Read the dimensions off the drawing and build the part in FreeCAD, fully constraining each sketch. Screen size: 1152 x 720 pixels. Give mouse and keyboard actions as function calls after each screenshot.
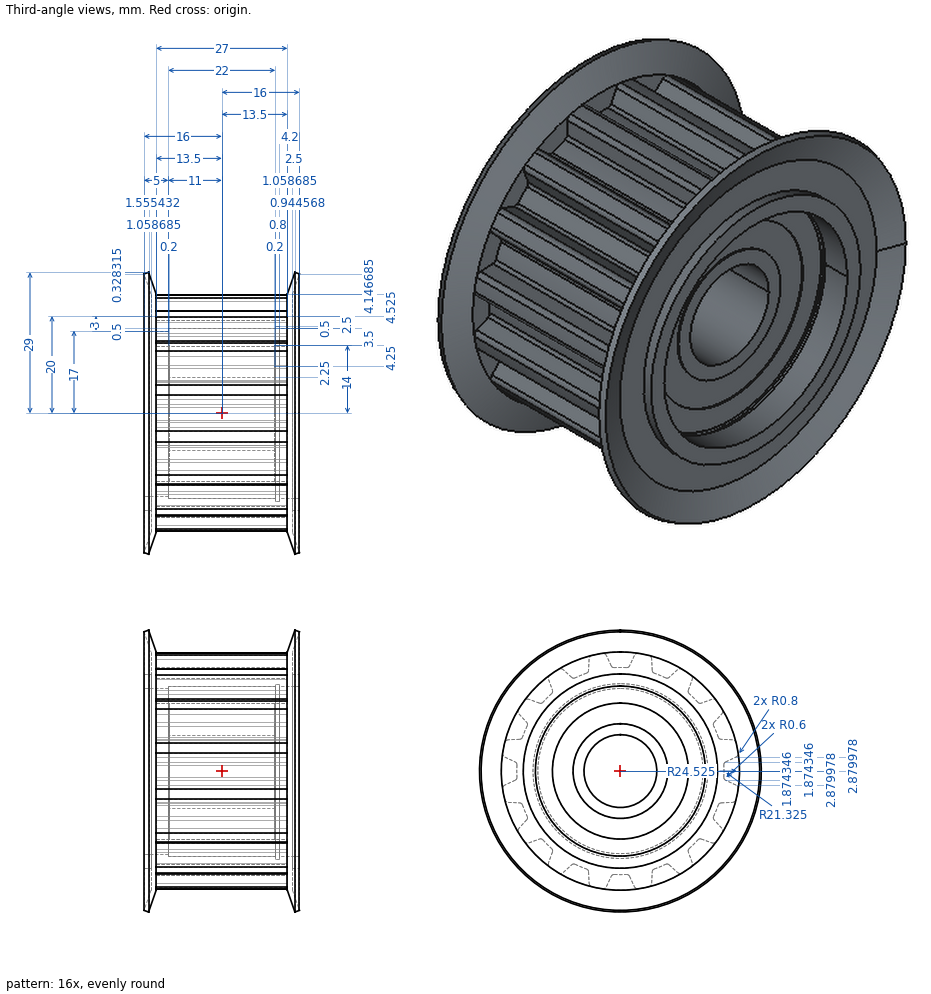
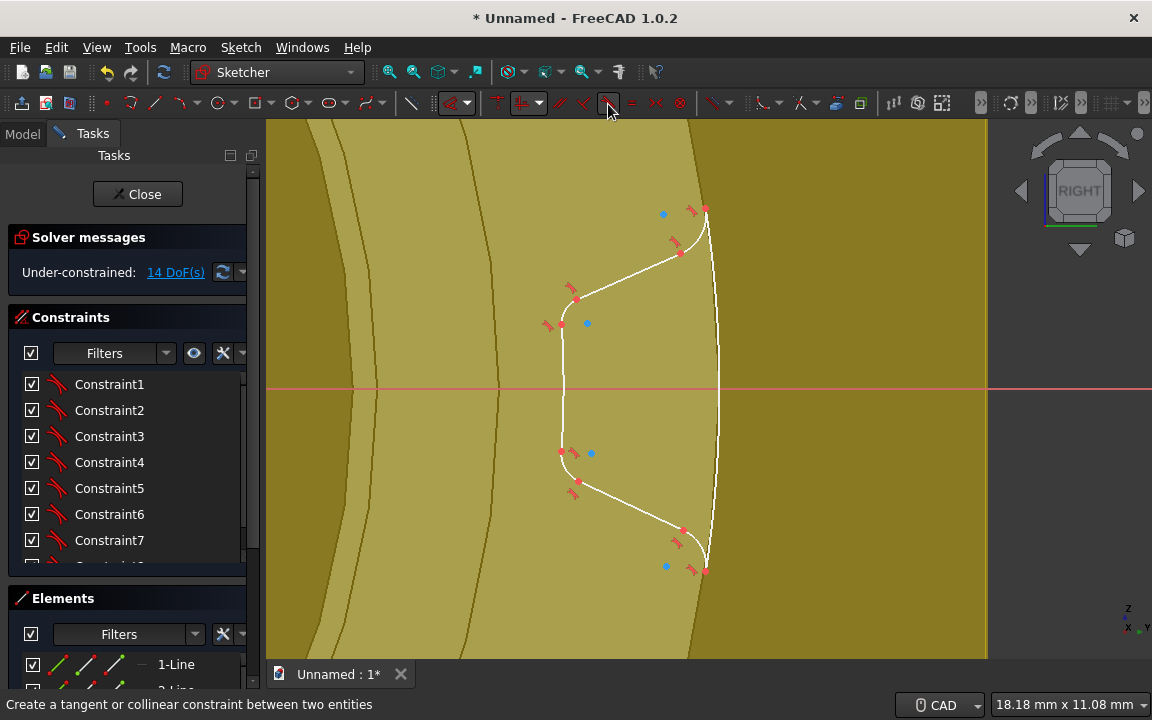
click(563, 414)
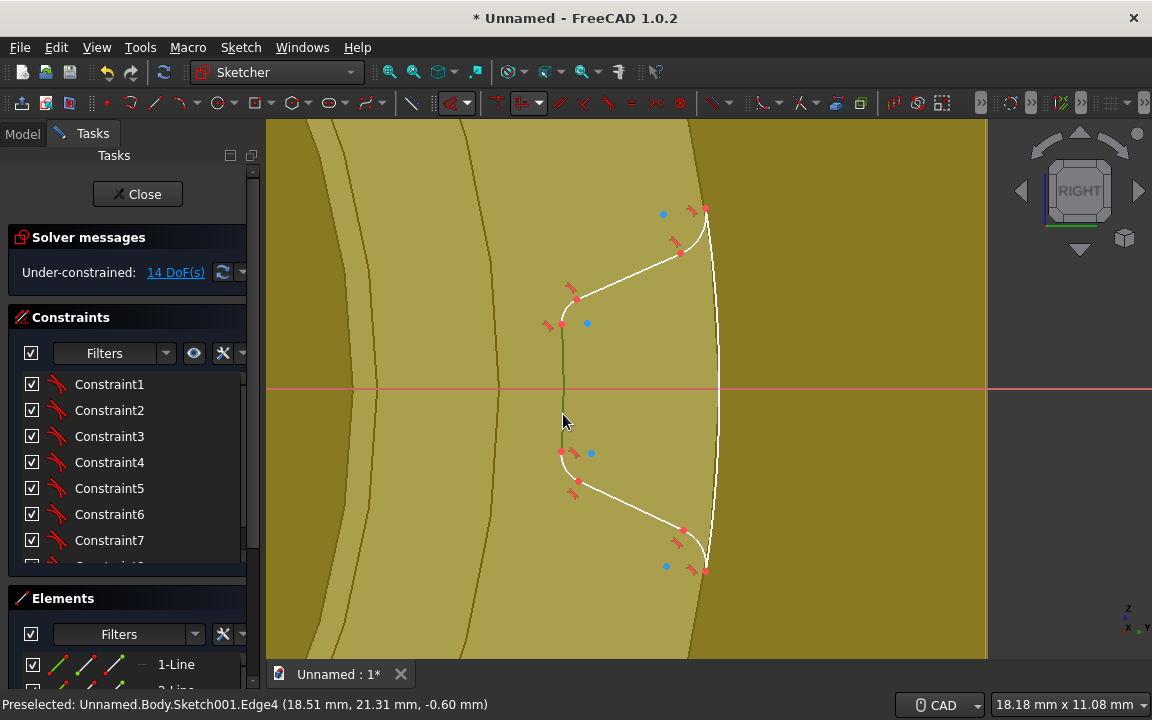
click(717, 463)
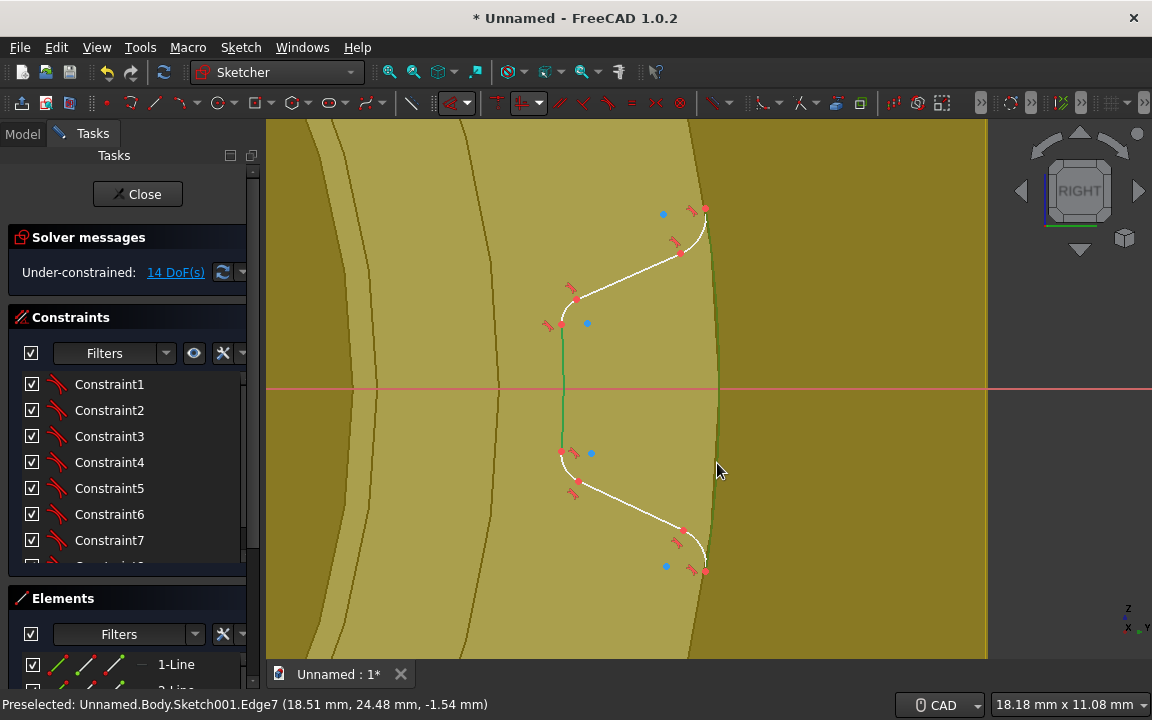
click(498, 104)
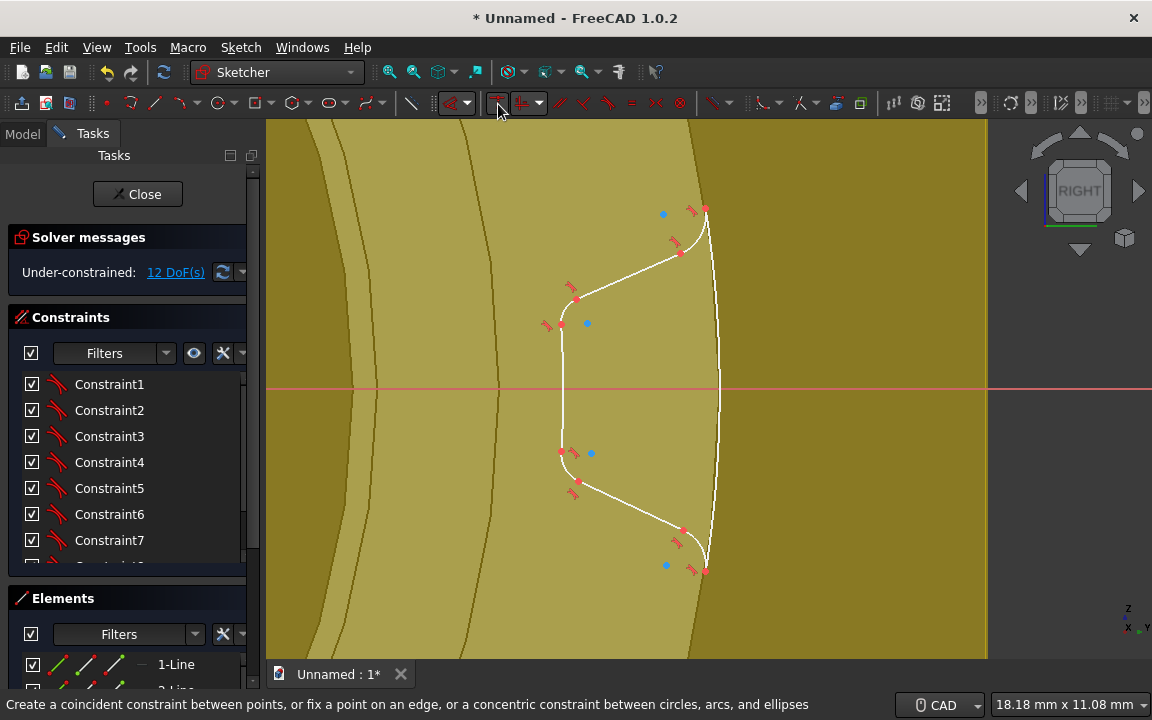
scroll(987, 389, down, 4)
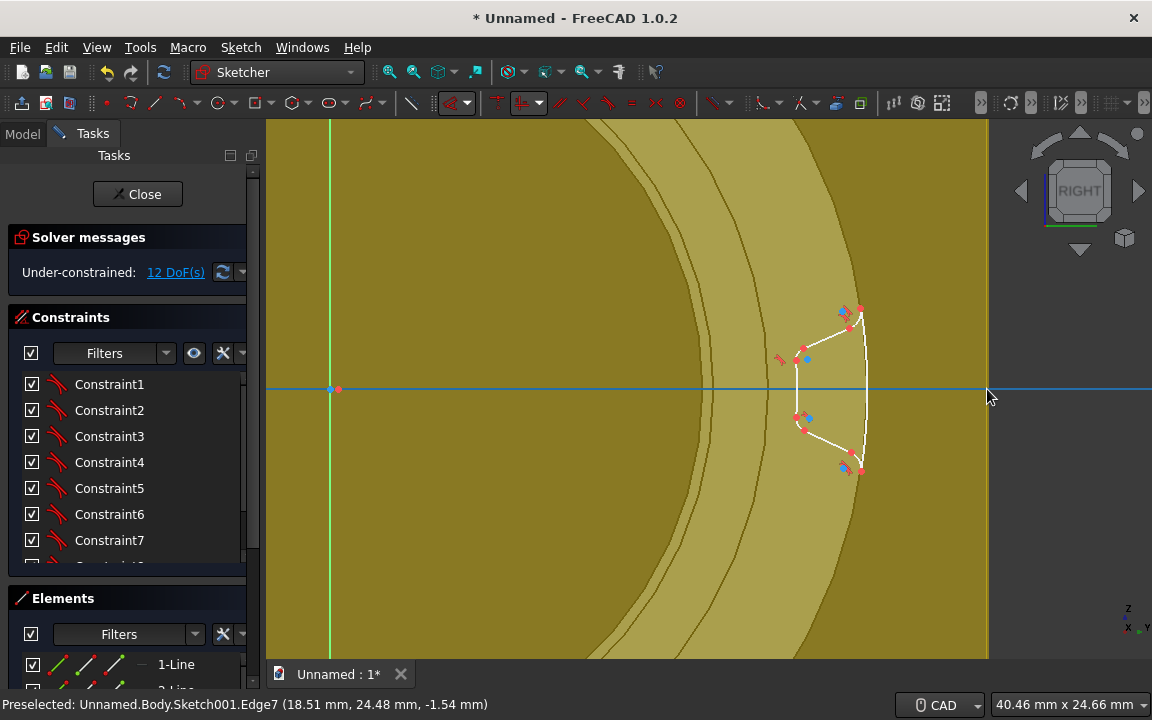
scroll(334, 390, up, 7)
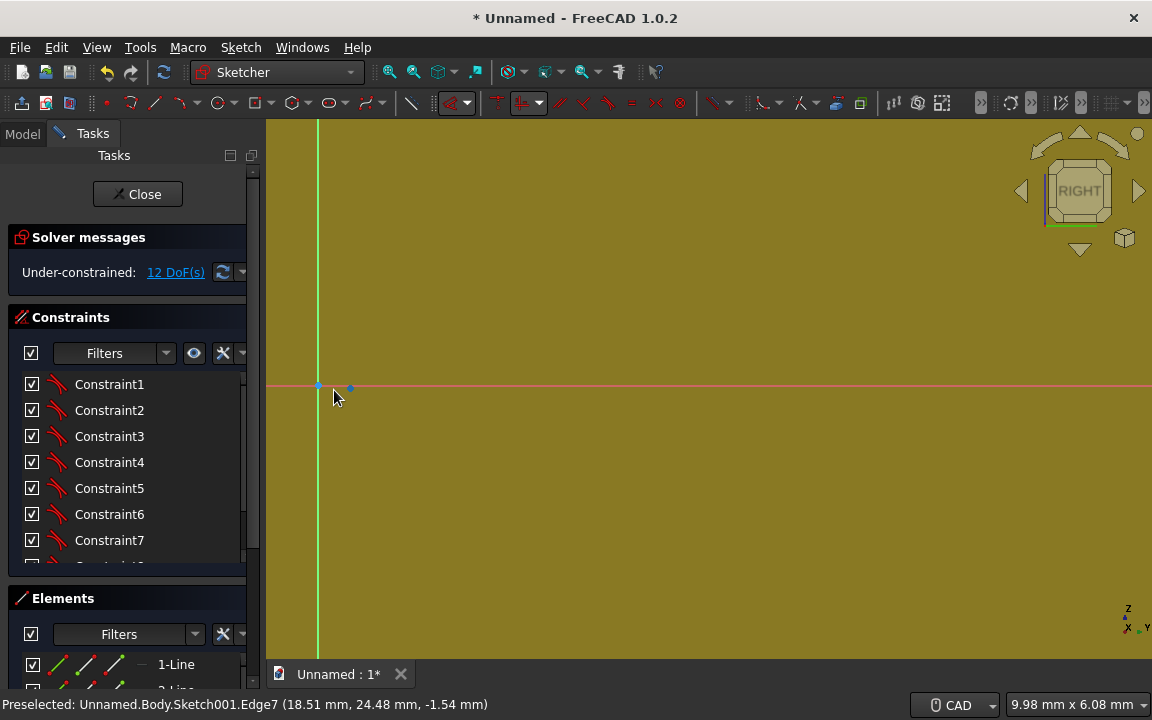
drag(308, 376, 360, 398)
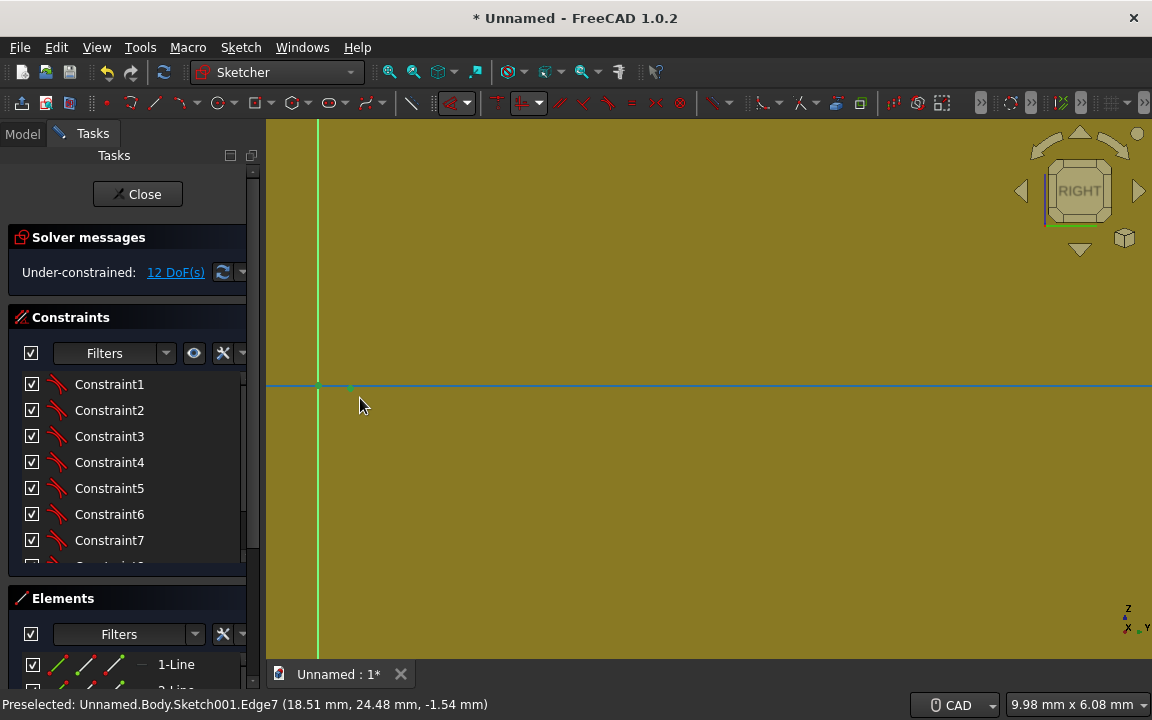
click(498, 104)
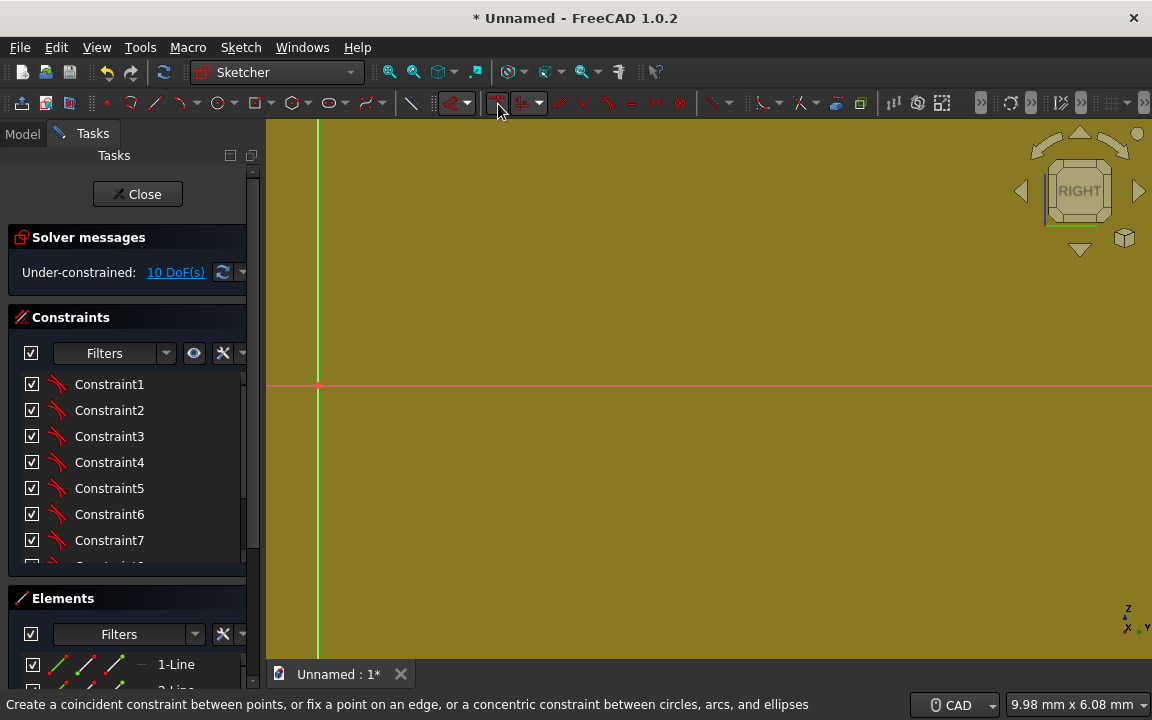
scroll(294, 390, down, 6)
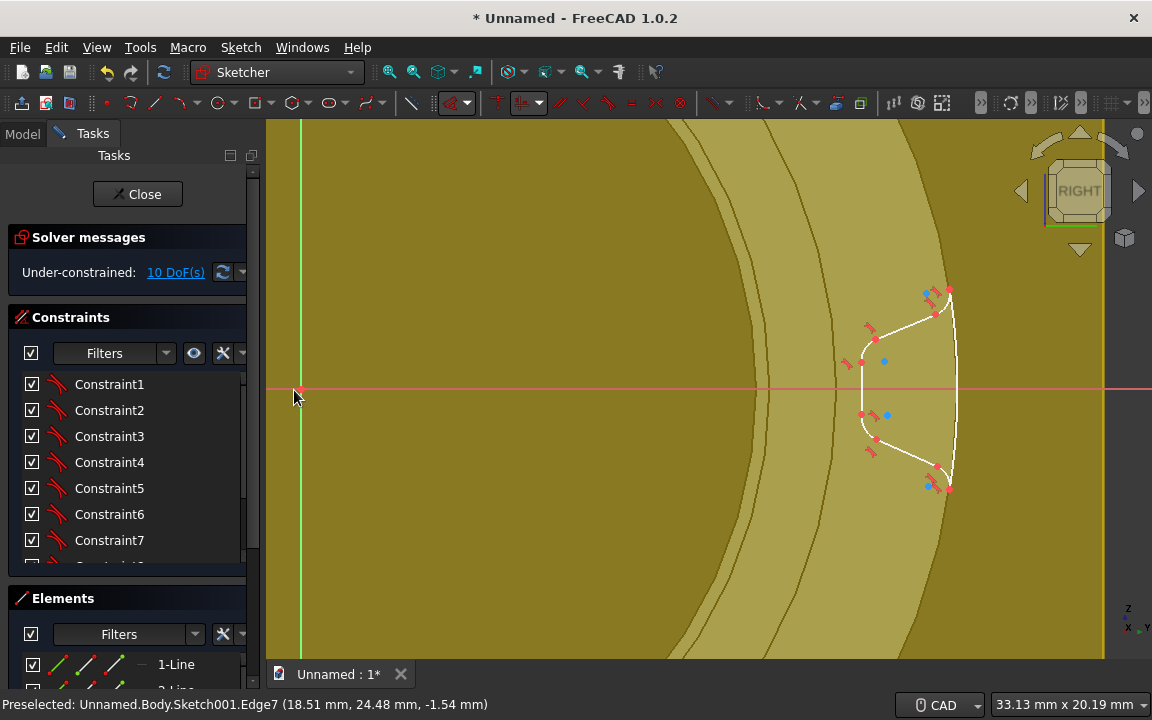
scroll(987, 389, up, 3)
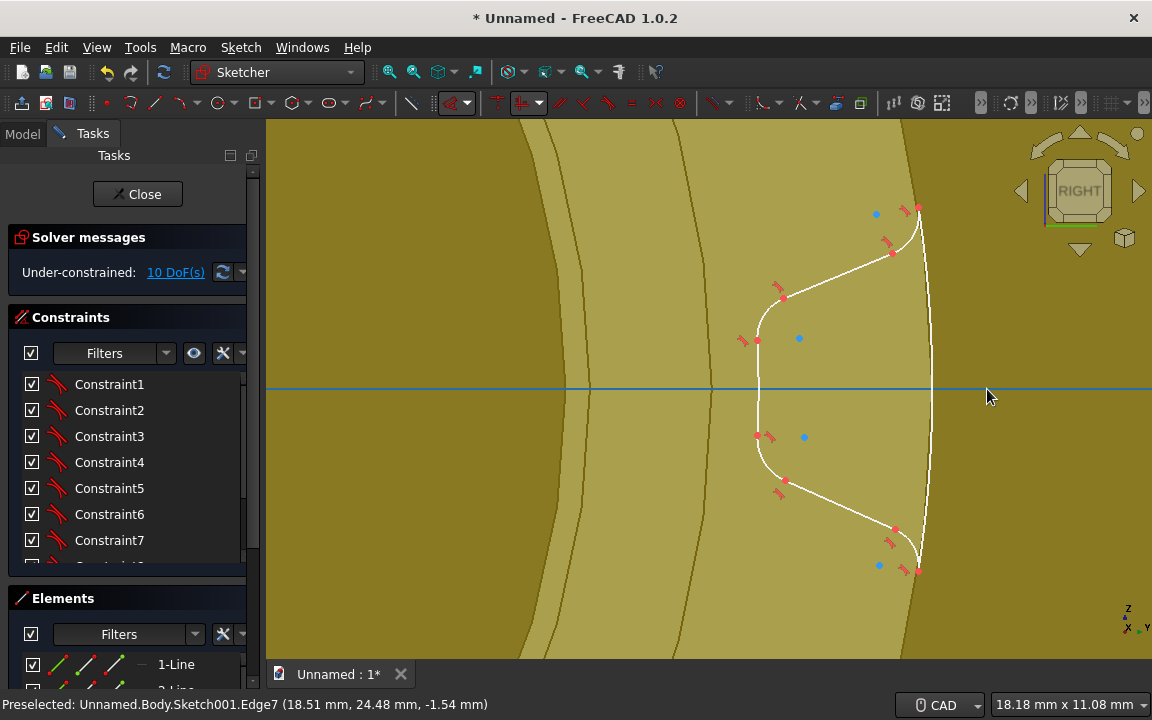
click(760, 452)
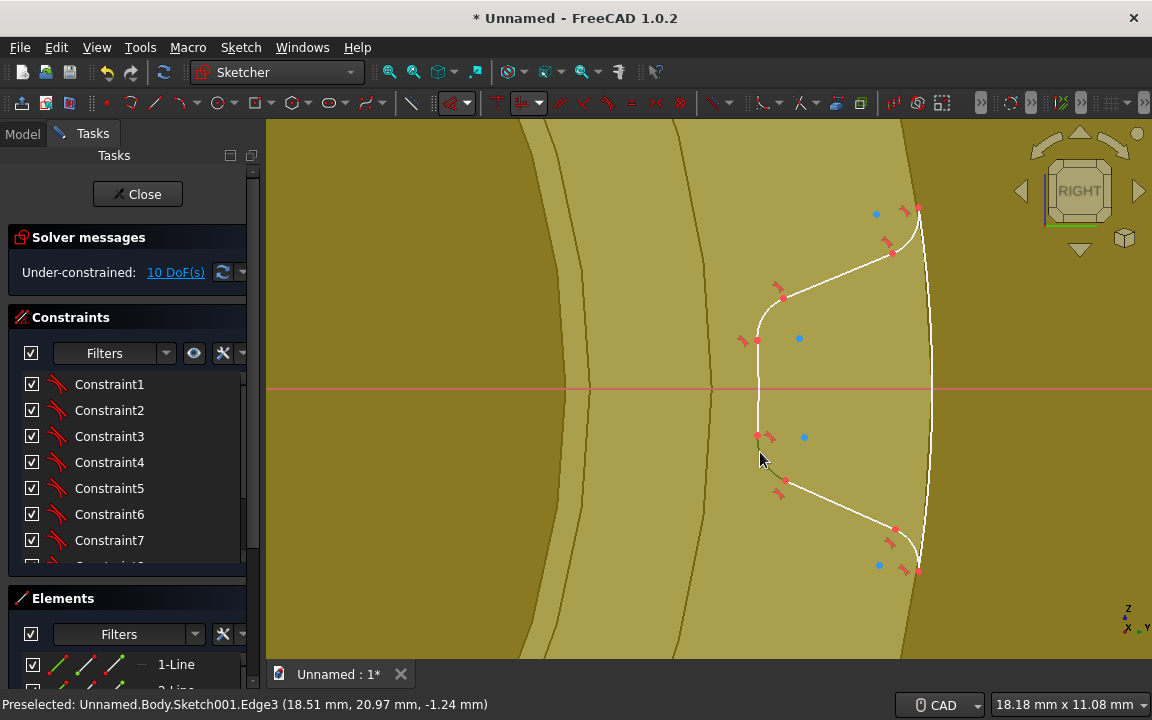
click(771, 307)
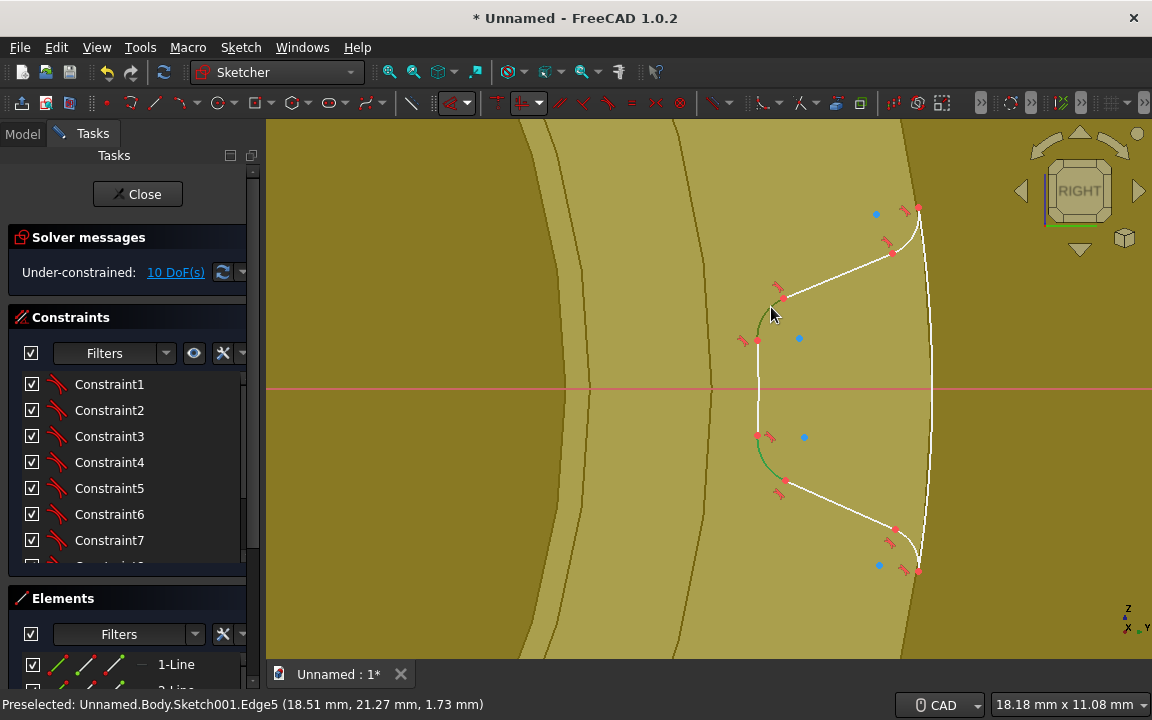
click(632, 104)